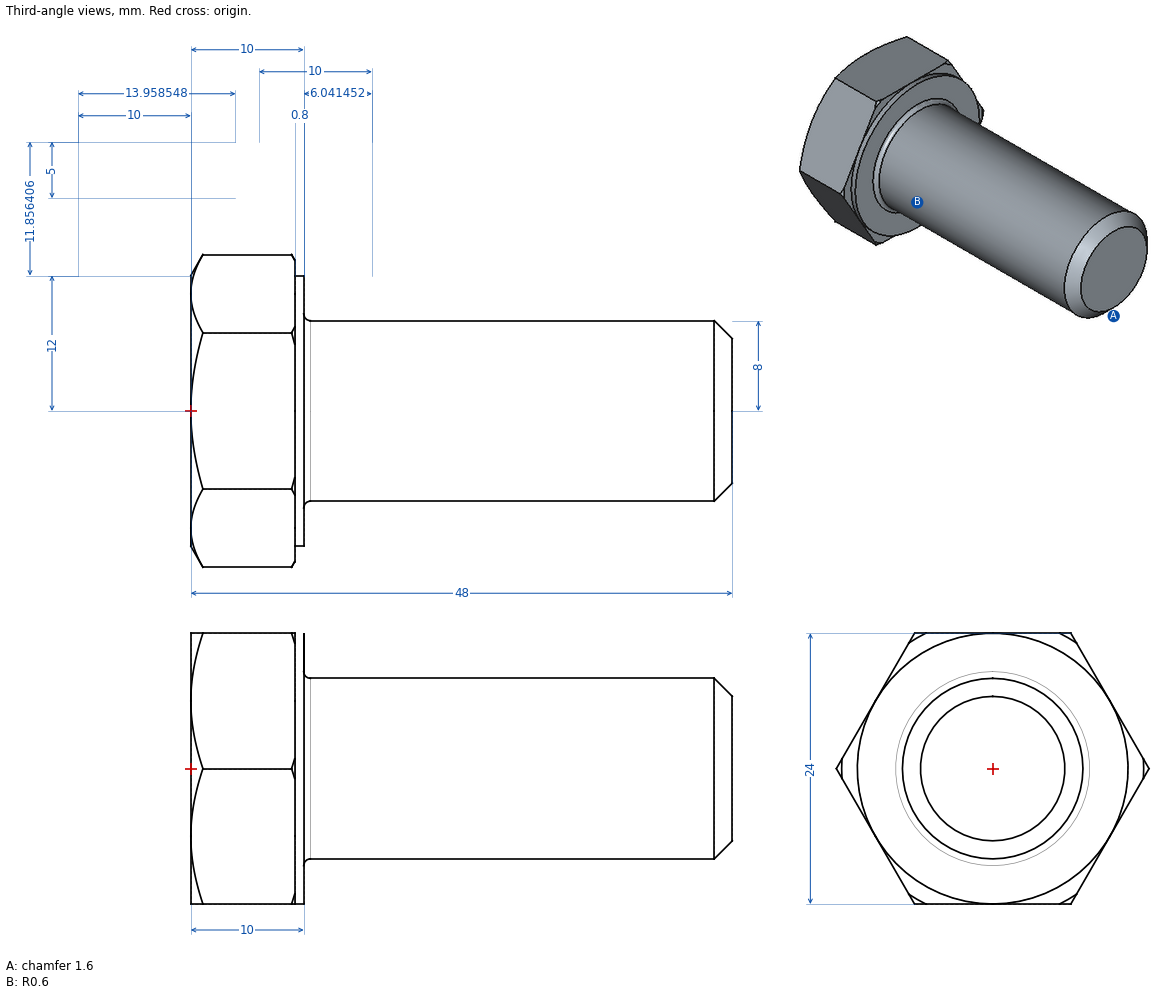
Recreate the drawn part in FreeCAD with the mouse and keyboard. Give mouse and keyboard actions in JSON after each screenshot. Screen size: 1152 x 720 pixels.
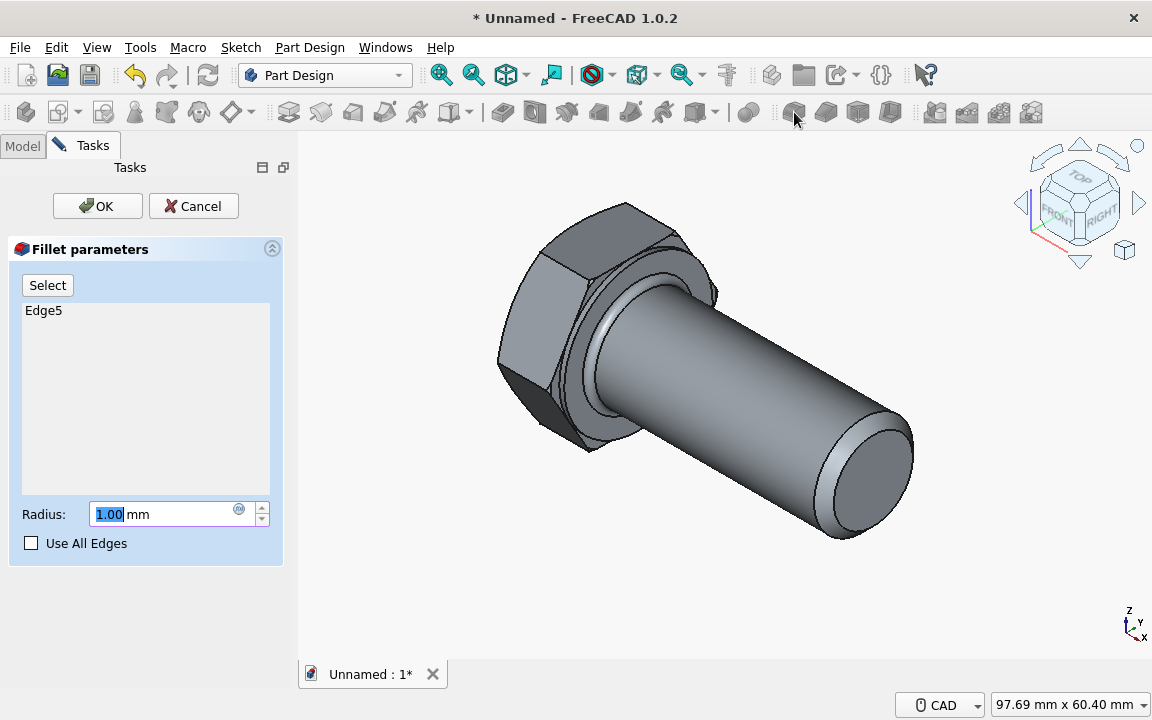
{"action": "type", "text": "0.6"}
{"action": "key", "text": "Tab"}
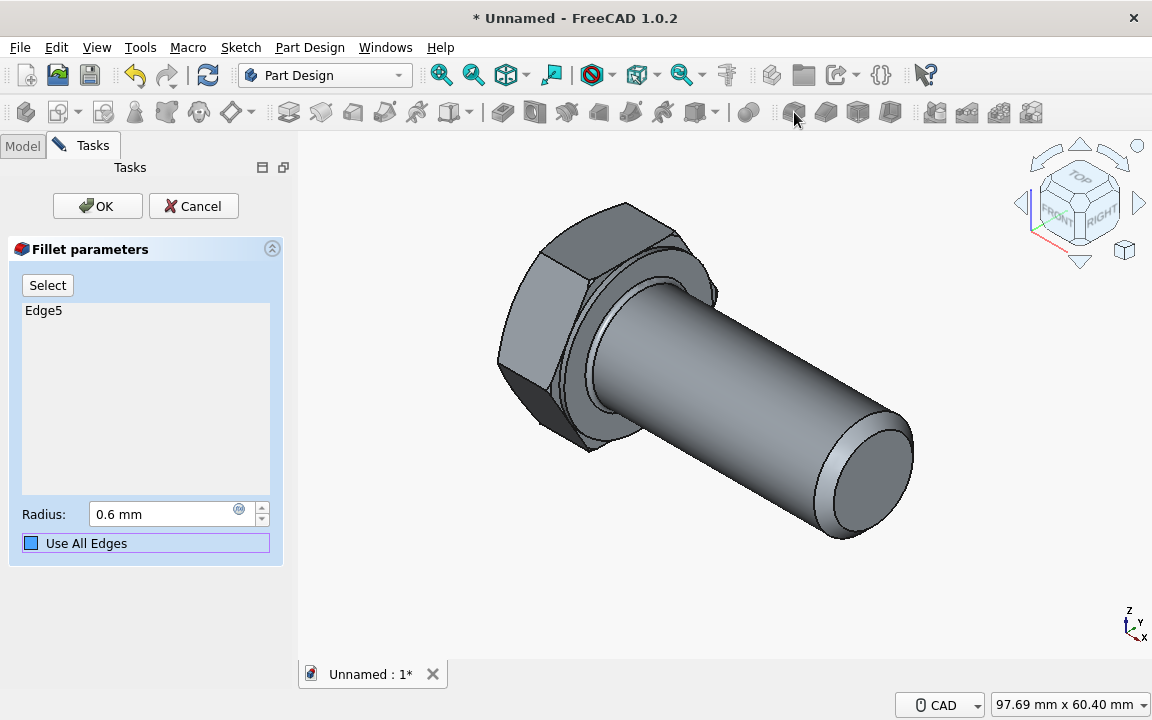
{"action": "left_click", "coordinate": [98, 206]}